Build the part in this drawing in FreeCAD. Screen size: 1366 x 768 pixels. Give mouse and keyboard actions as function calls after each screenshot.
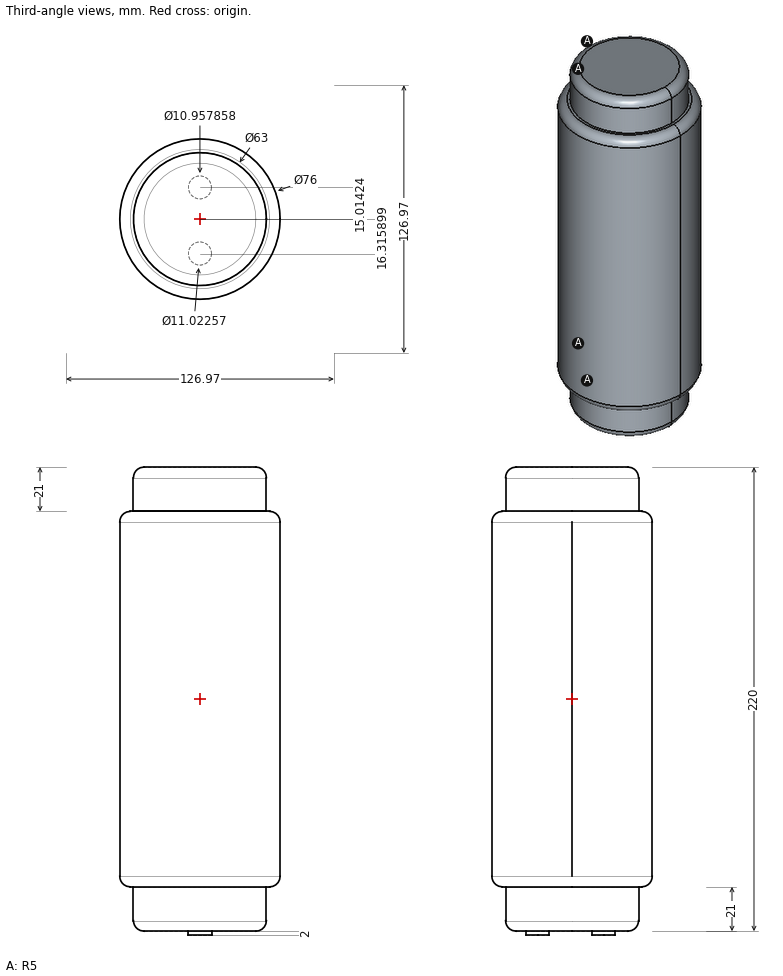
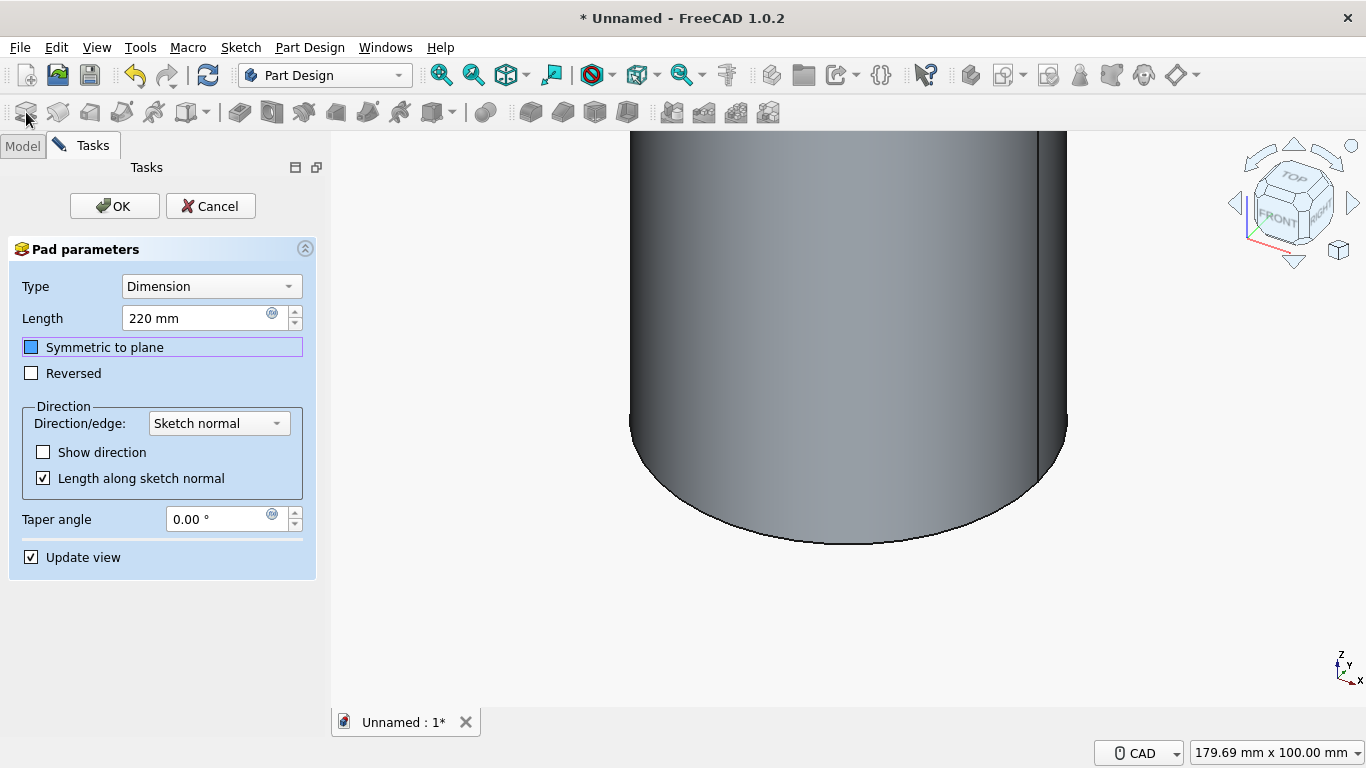
click(30, 347)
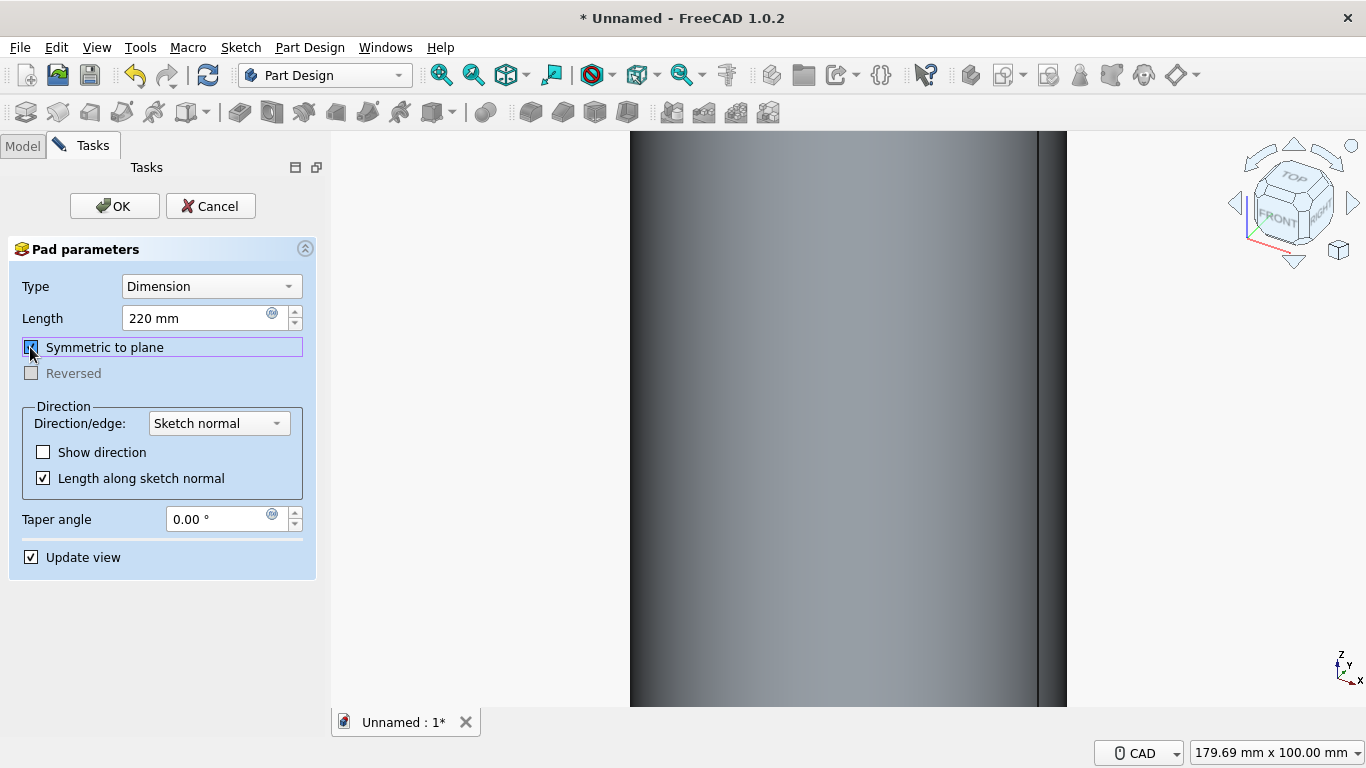
click(115, 206)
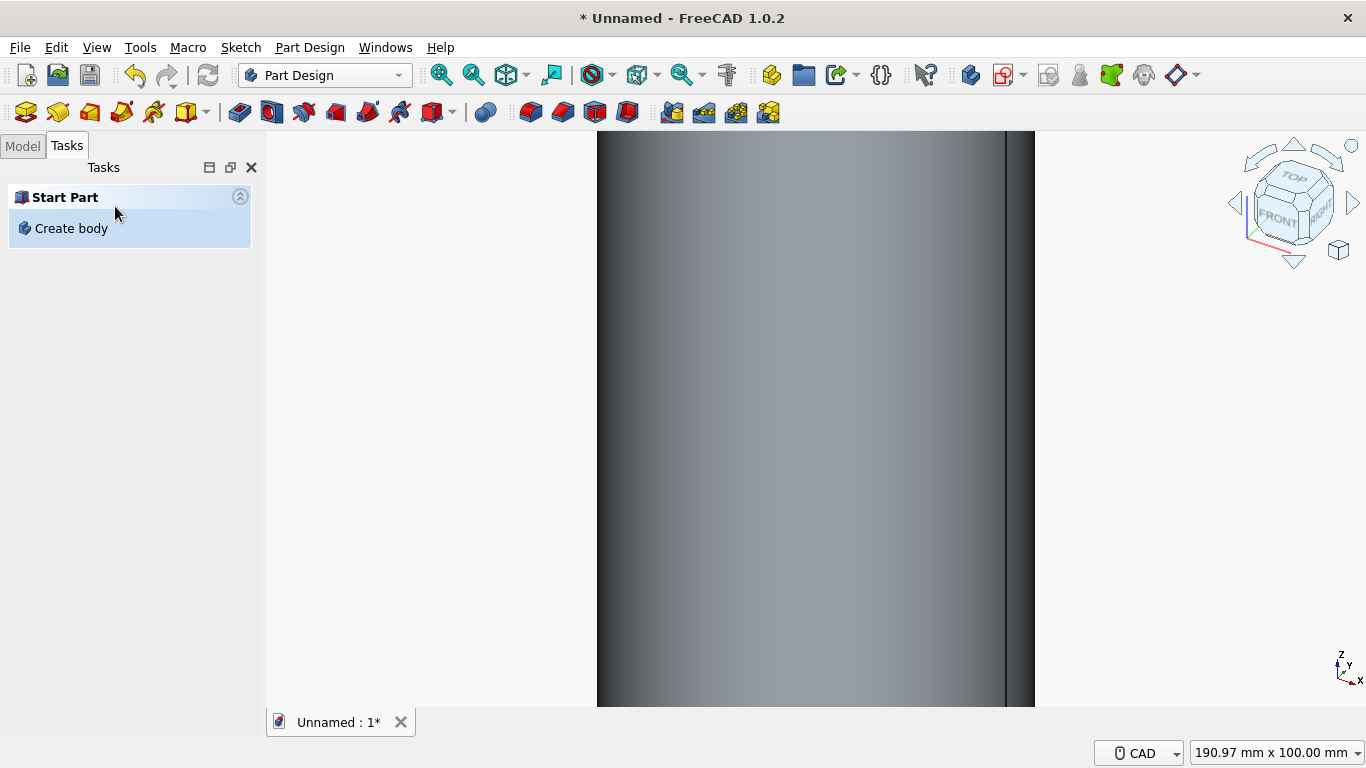
key(v)
key(f)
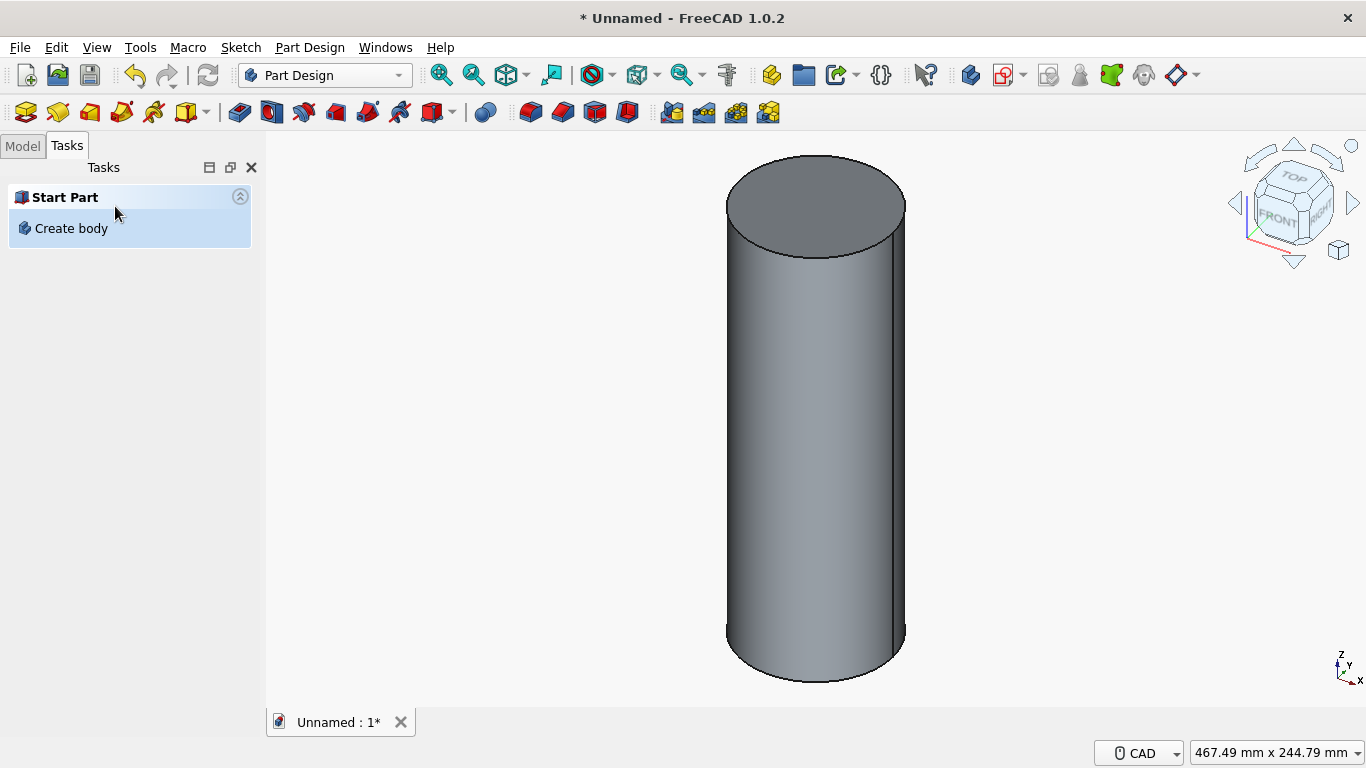
click(816, 206)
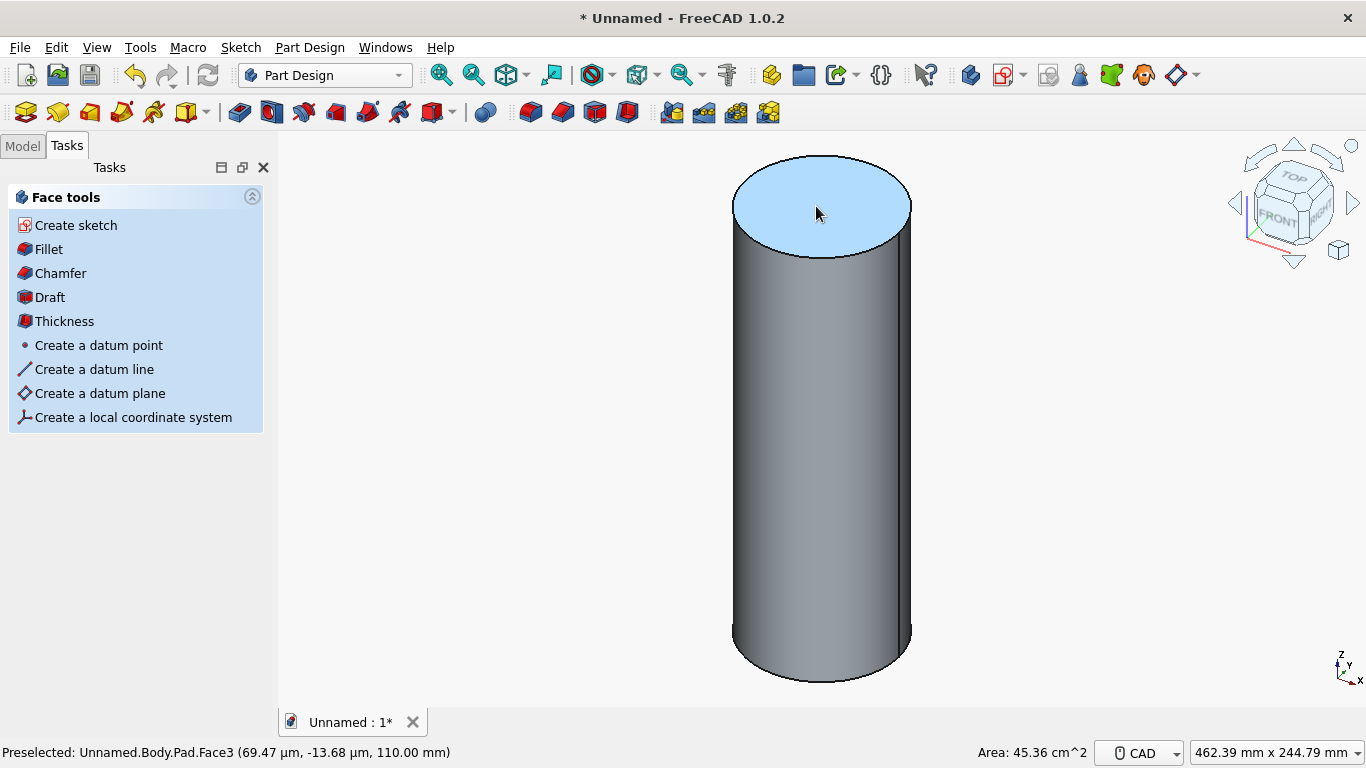
click(1004, 76)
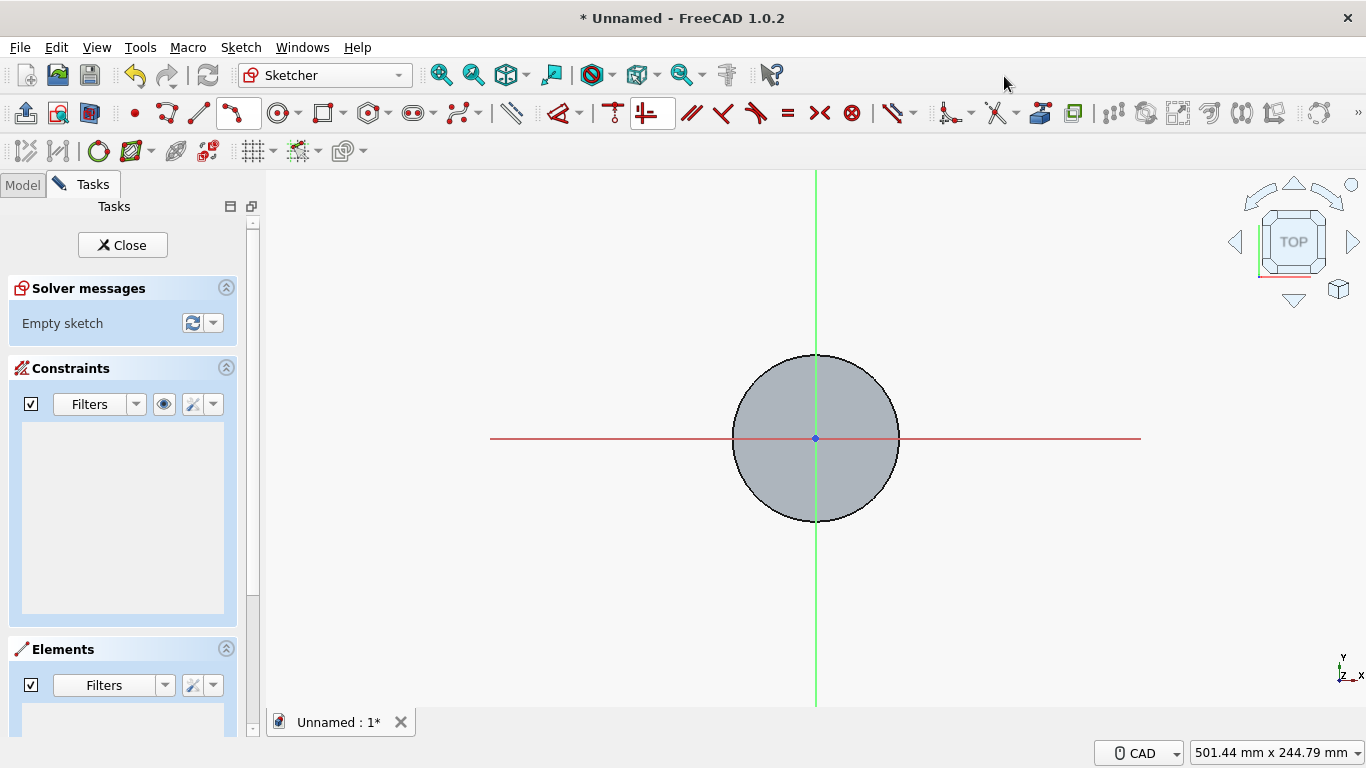
click(346, 114)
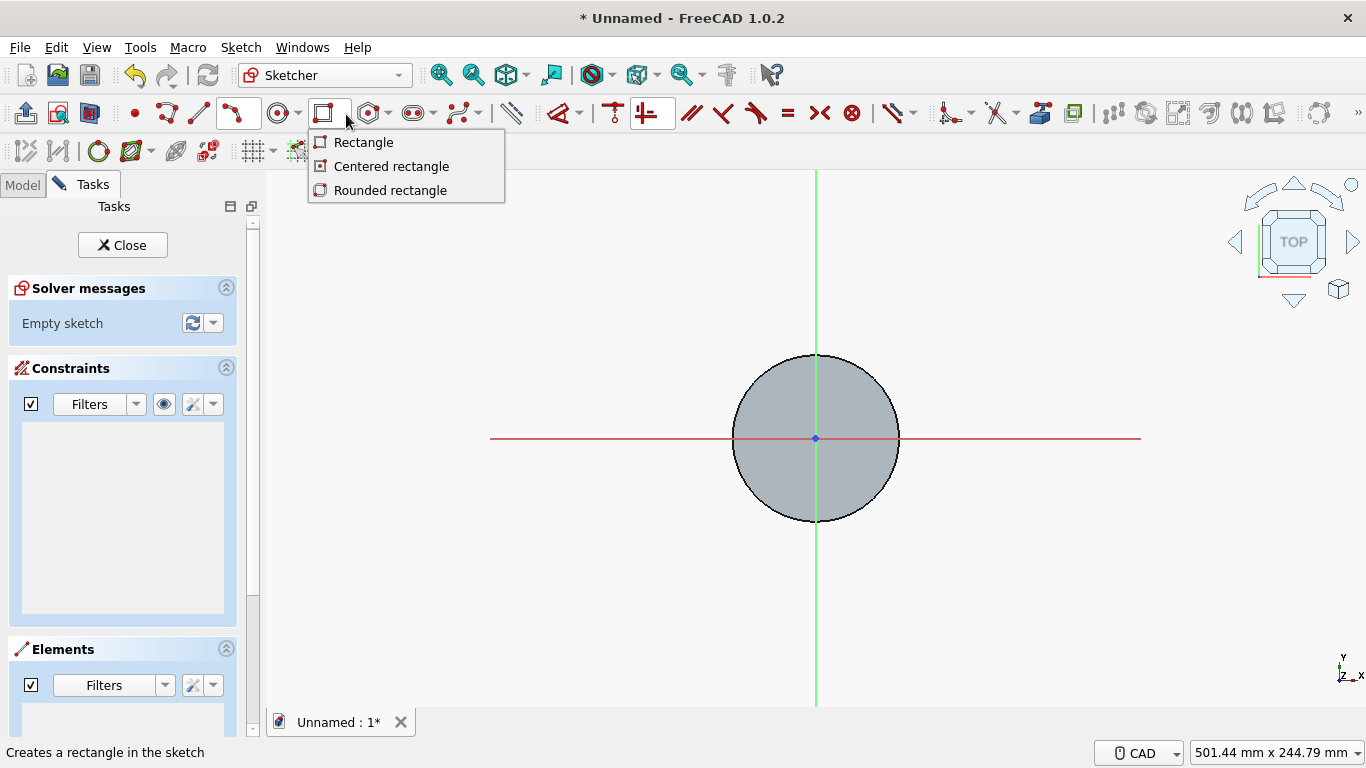
click(406, 166)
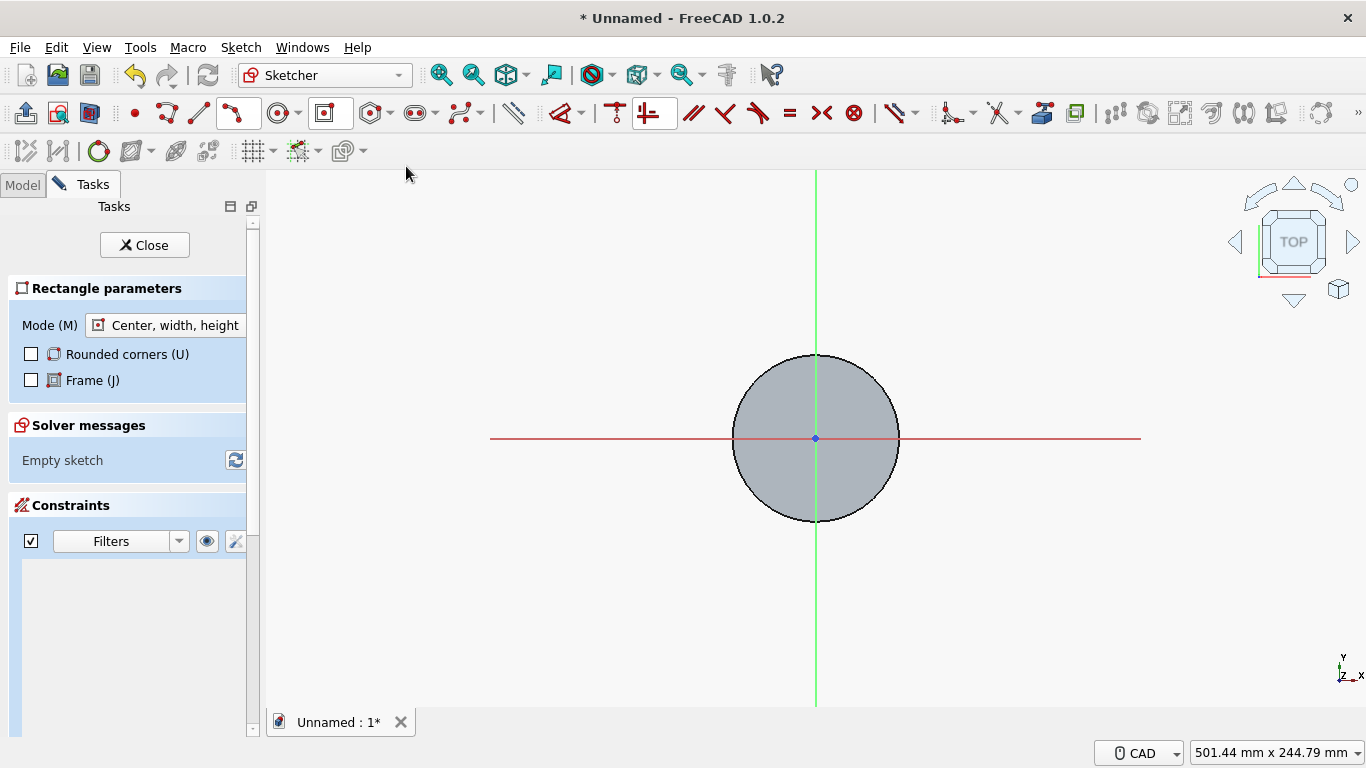
click(816, 438)
move(955, 299)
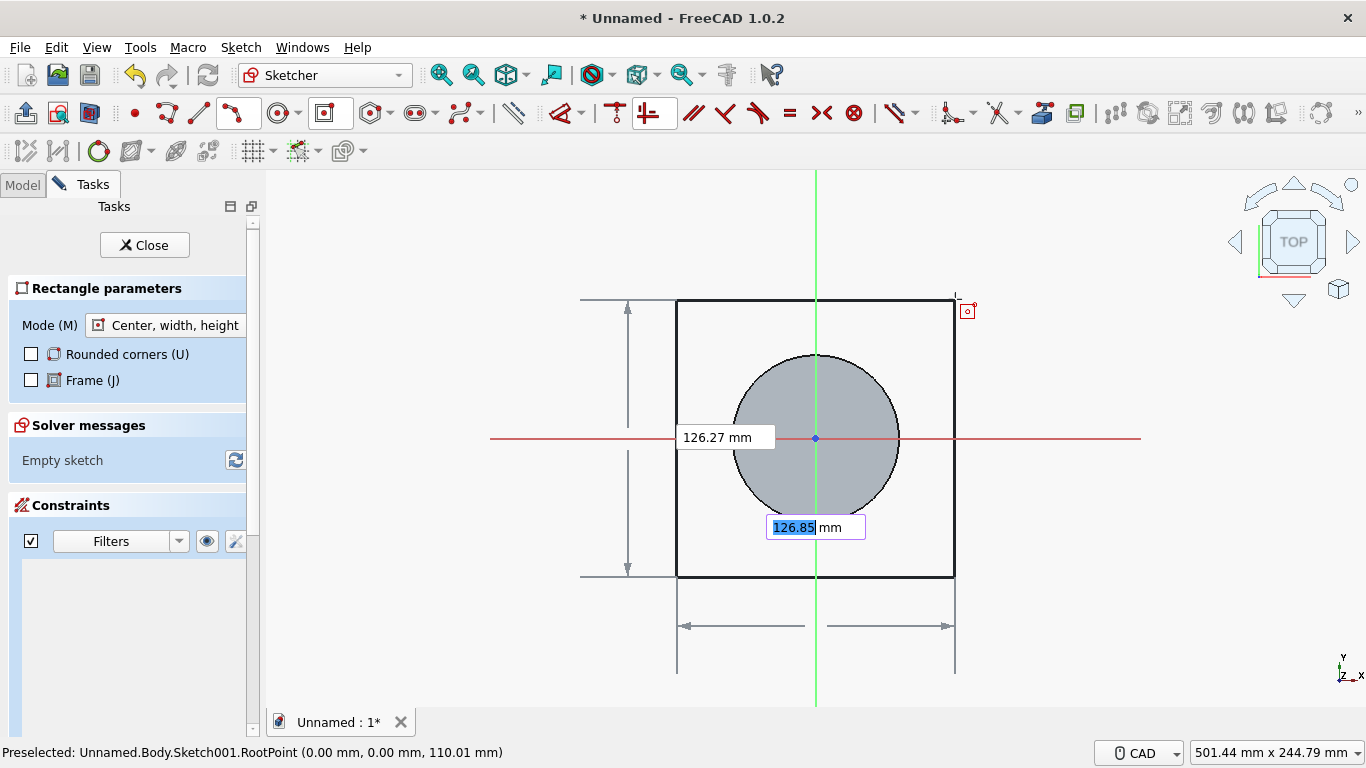
text(126.97)
key(Tab)
text(126.97)
key(Return)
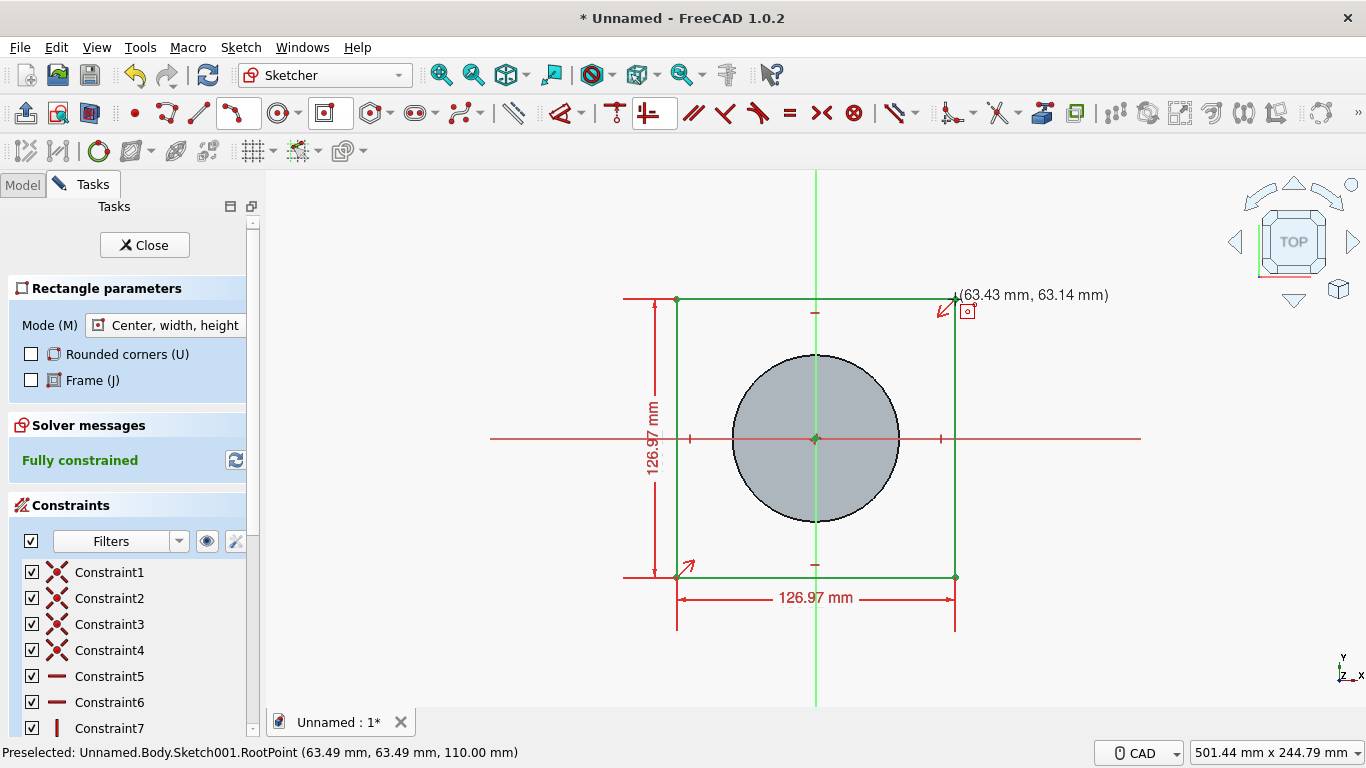
click(278, 114)